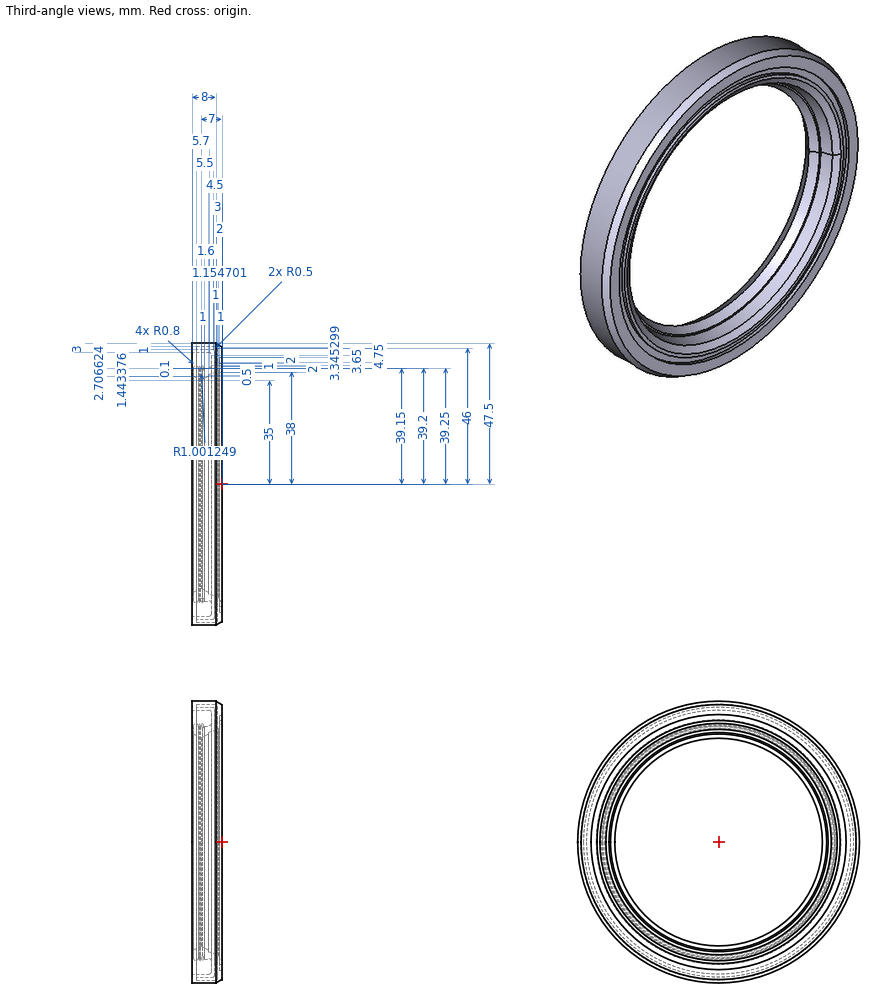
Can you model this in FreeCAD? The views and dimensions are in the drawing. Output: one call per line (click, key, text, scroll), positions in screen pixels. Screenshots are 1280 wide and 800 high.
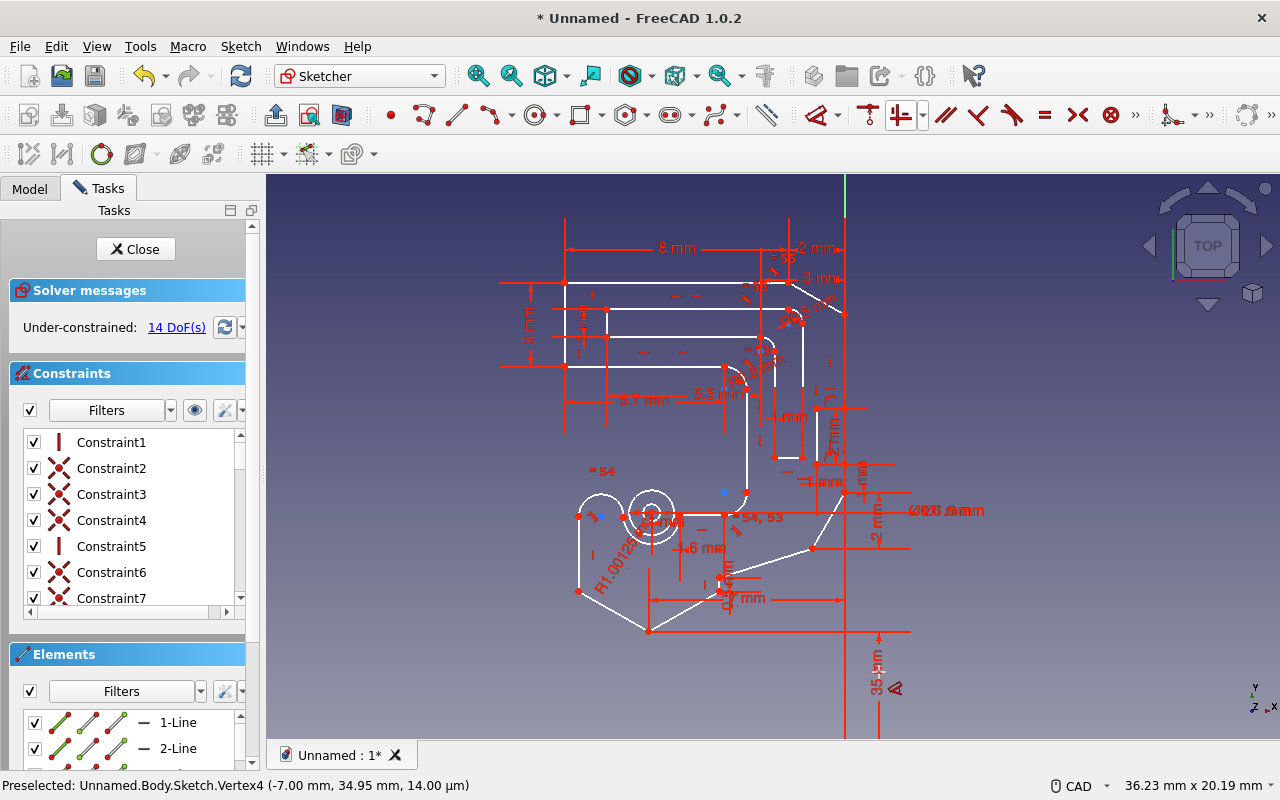
click(812, 549)
click(879, 630)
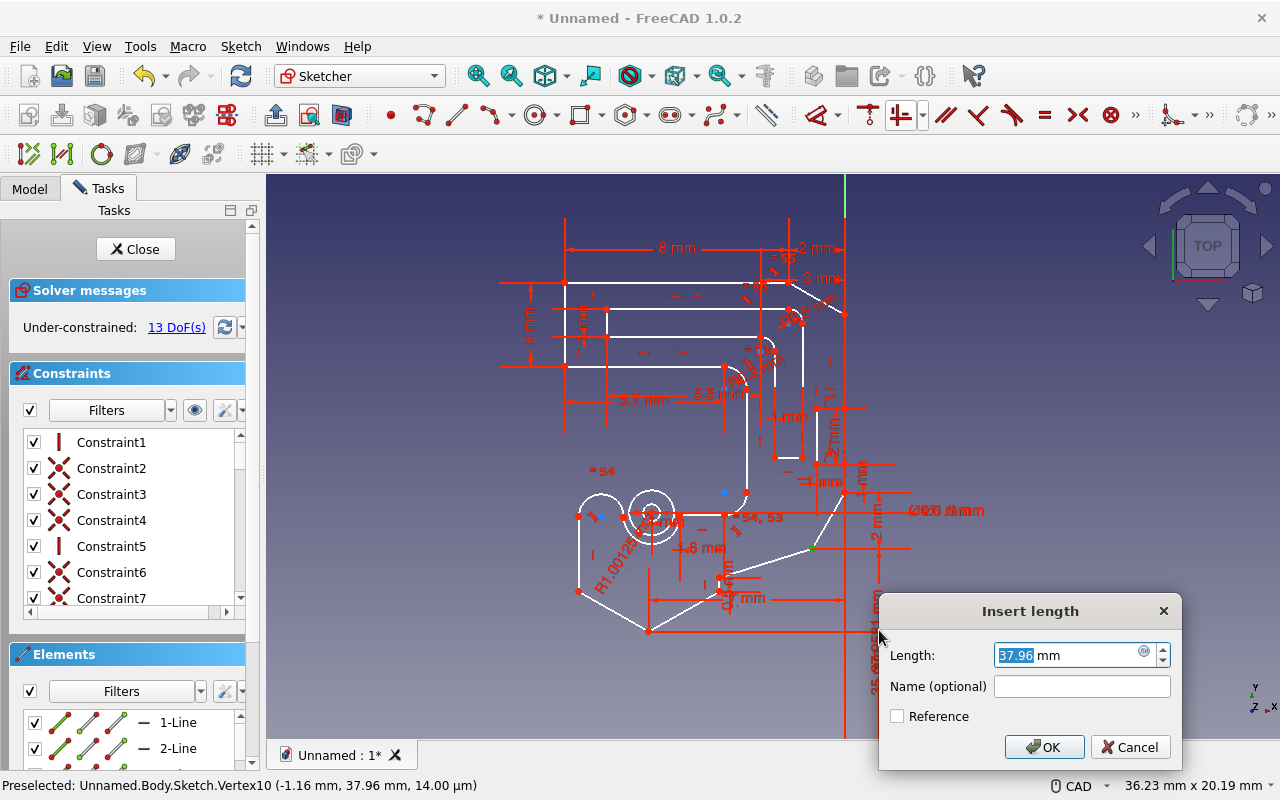
text(38)
key(Return)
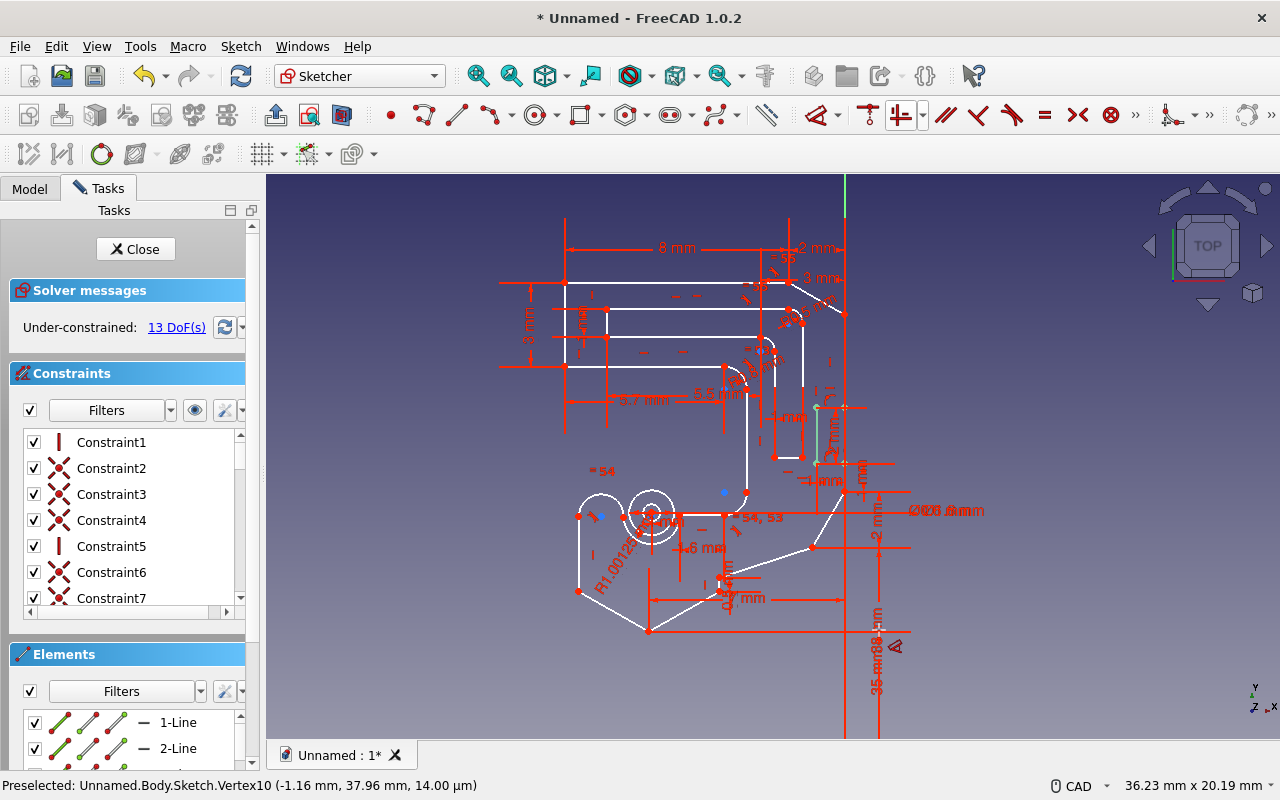
click(803, 323)
click(879, 606)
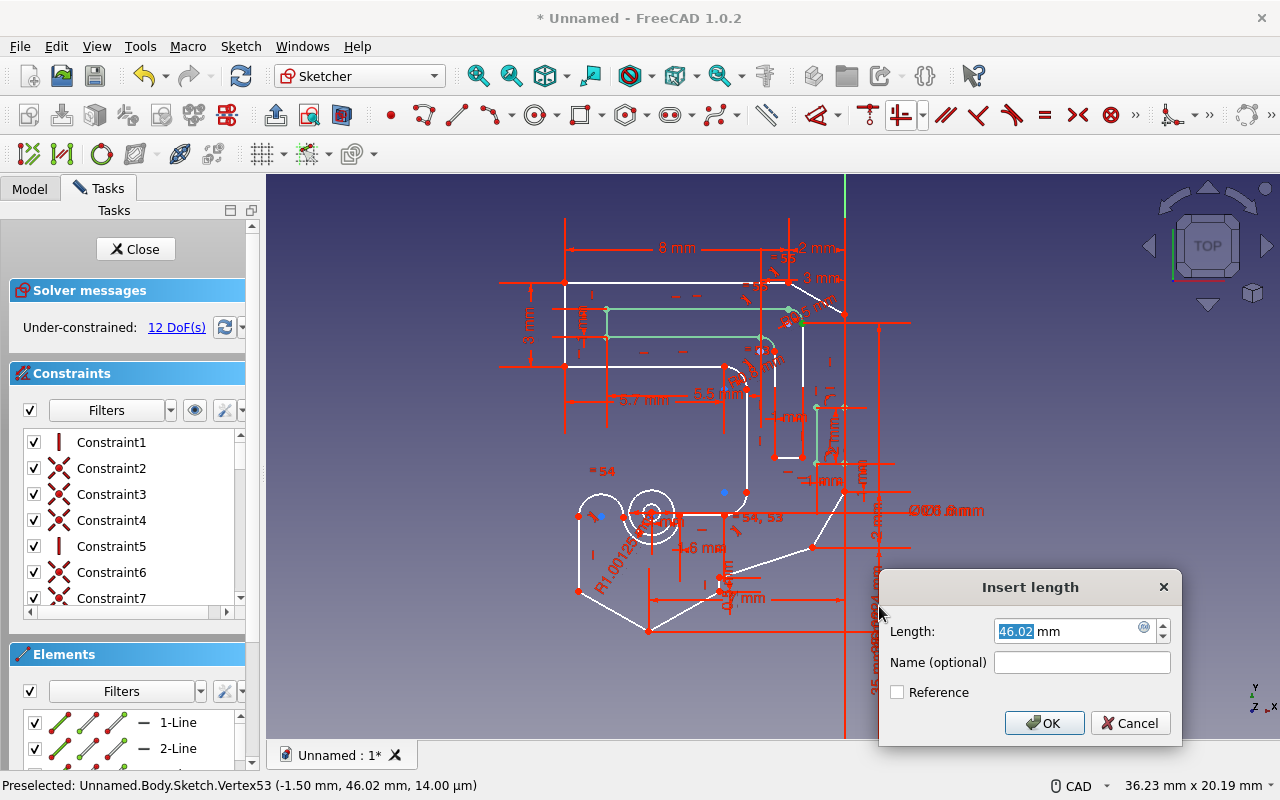
text(46)
key(Return)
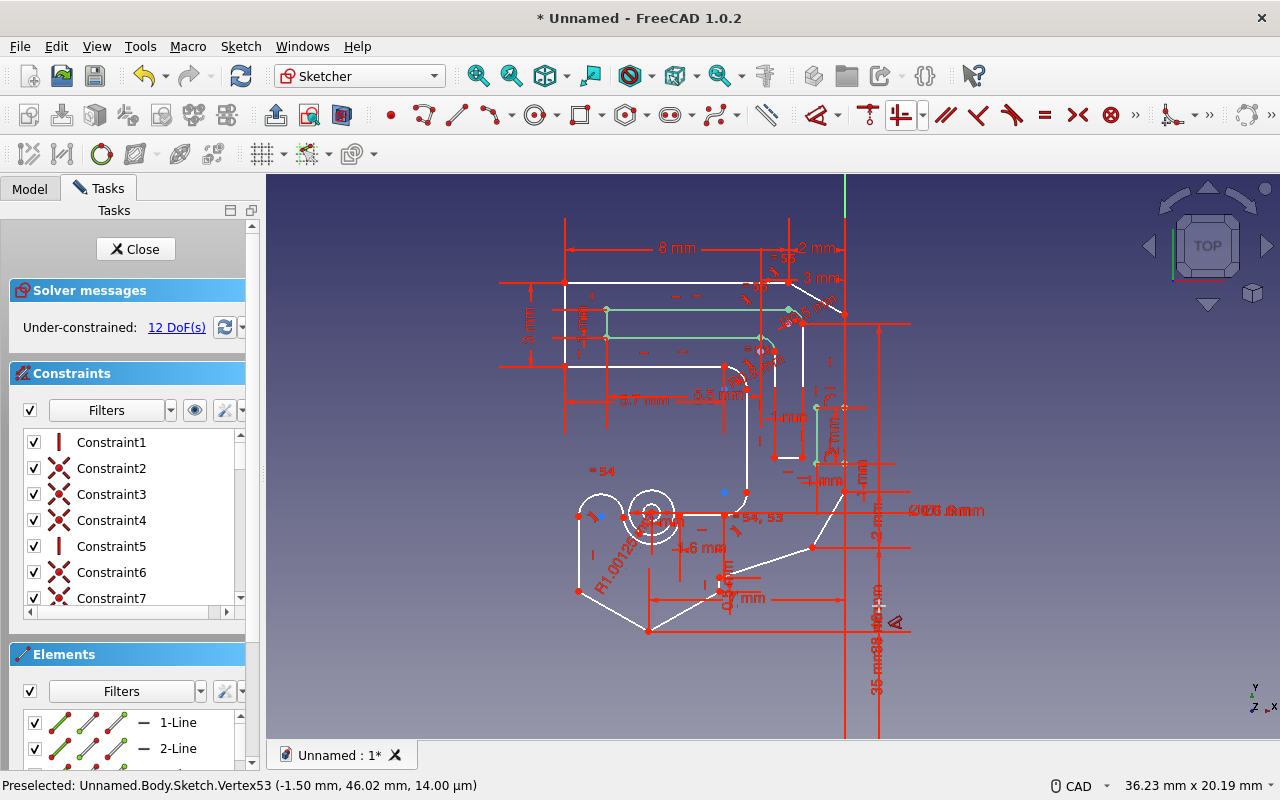
click(747, 420)
click(713, 441)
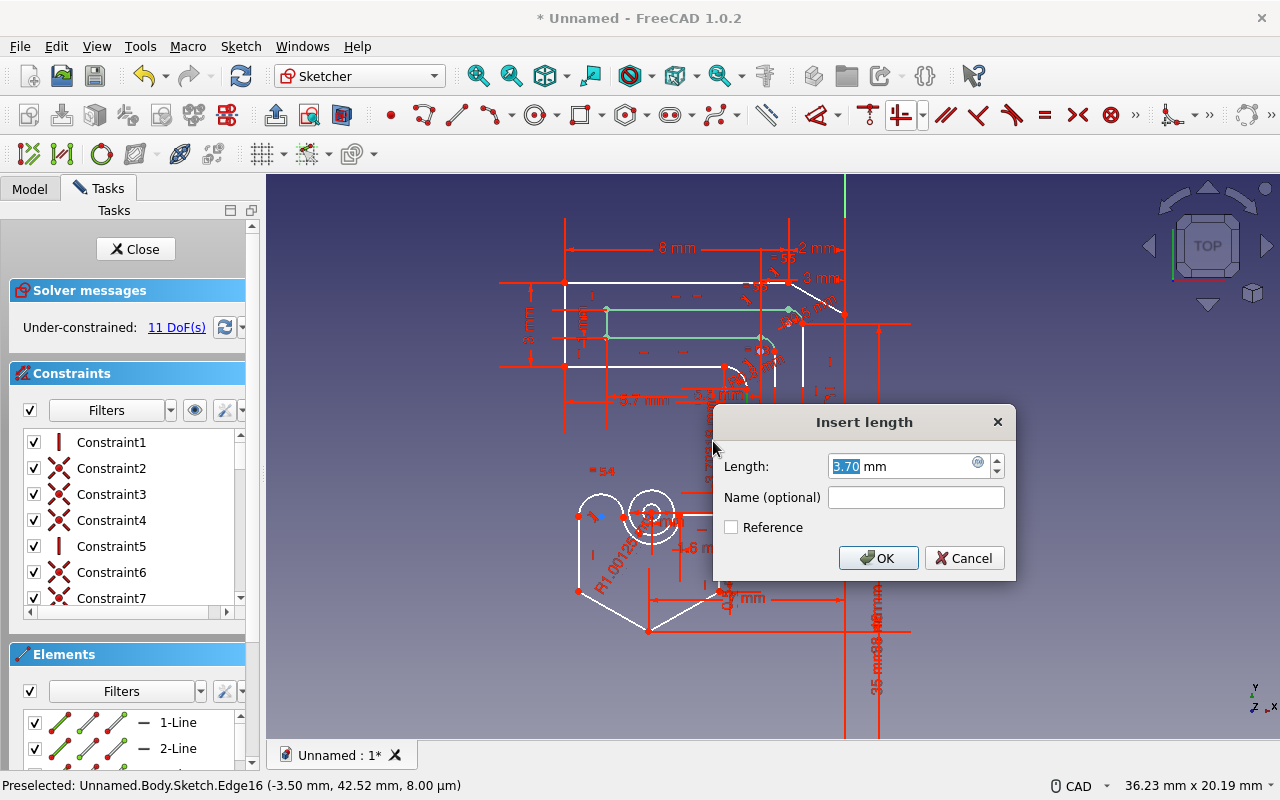
text(3.65)
key(Return)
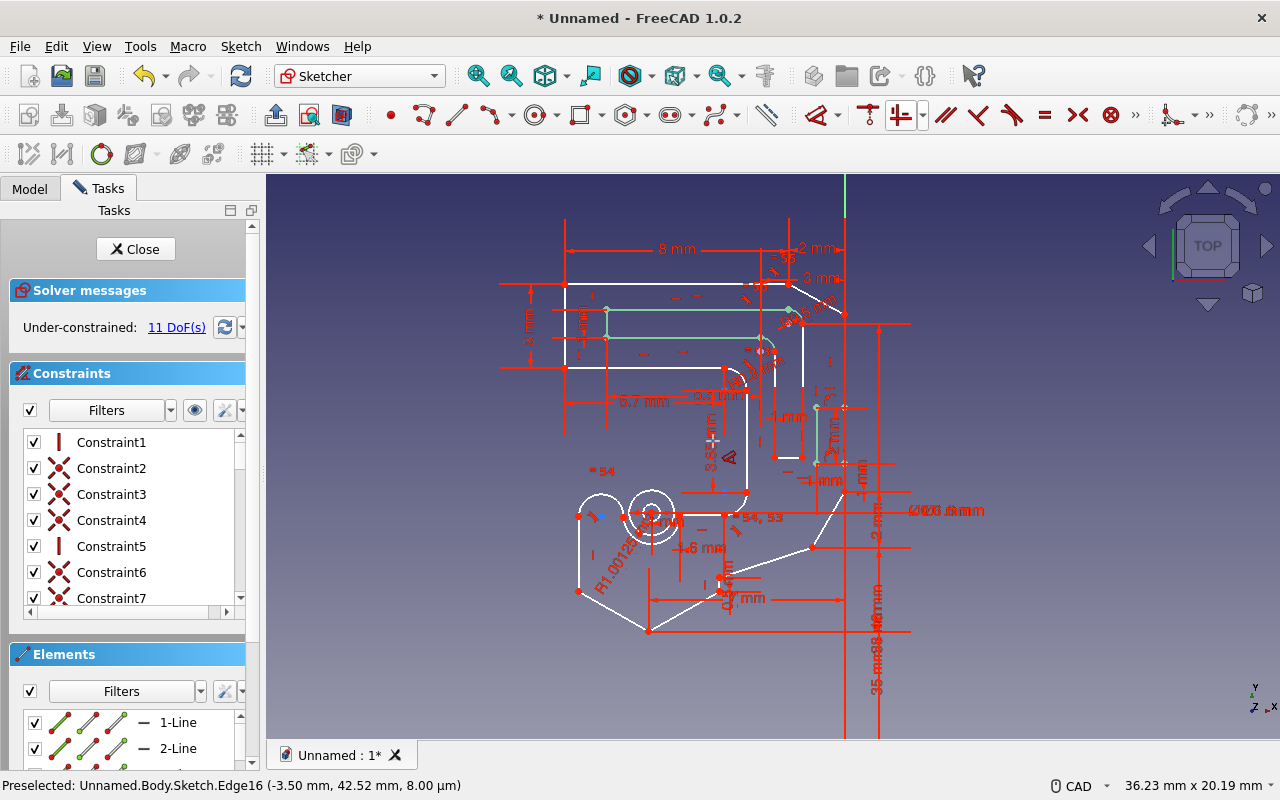
click(803, 364)
click(861, 391)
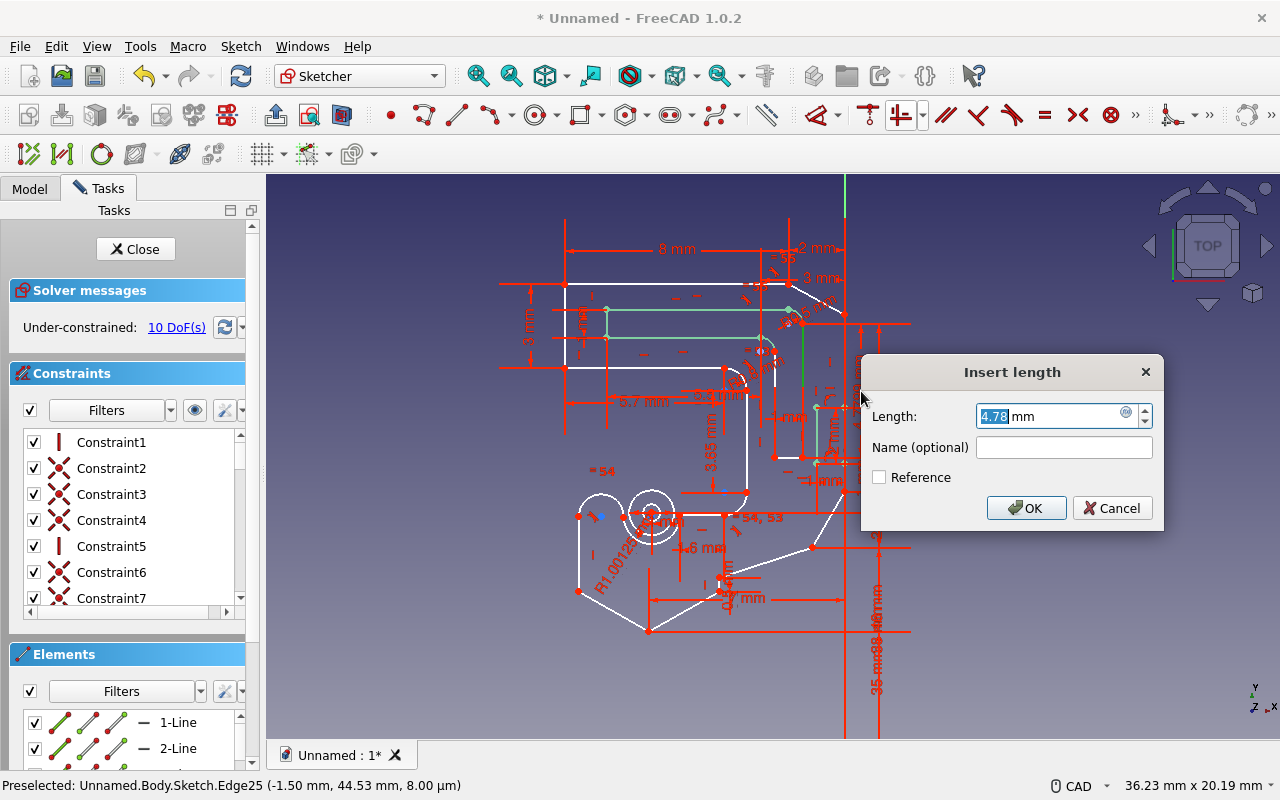
text(4.75)
key(Return)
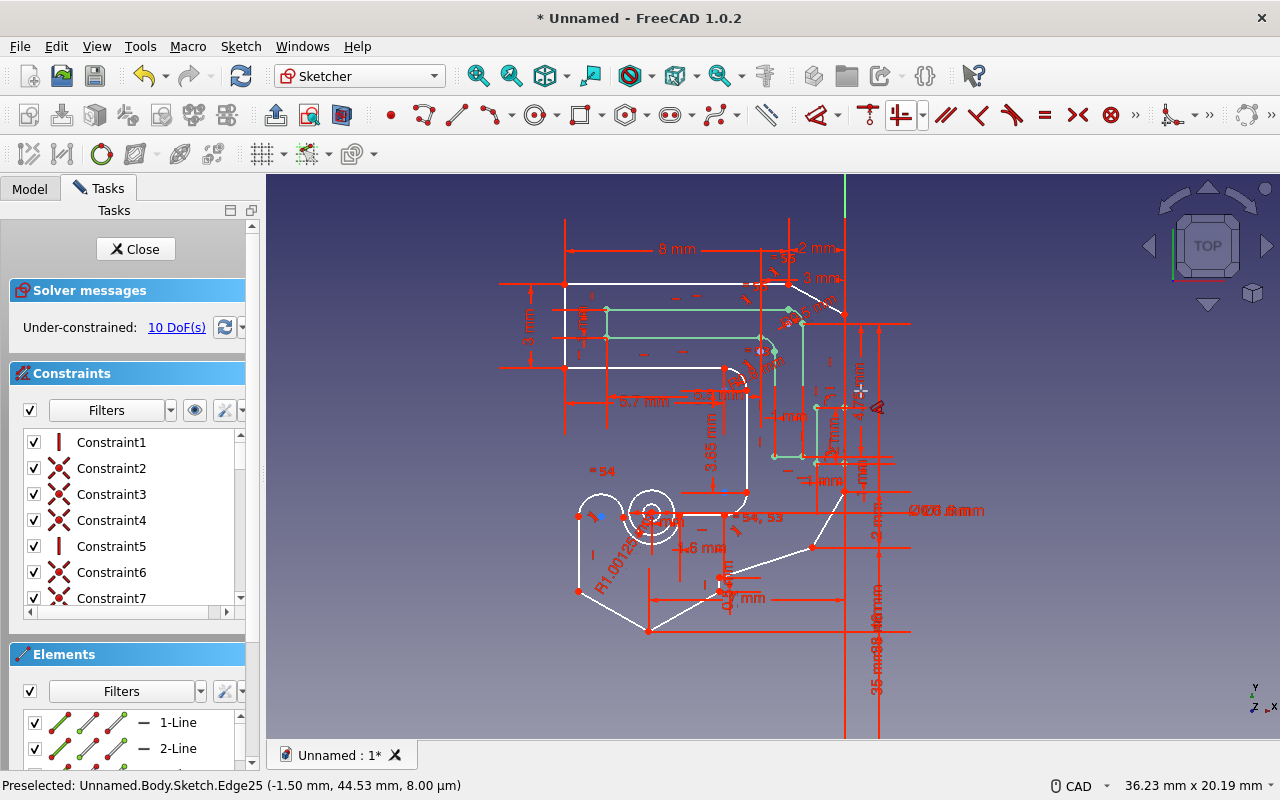
click(719, 592)
click(826, 558)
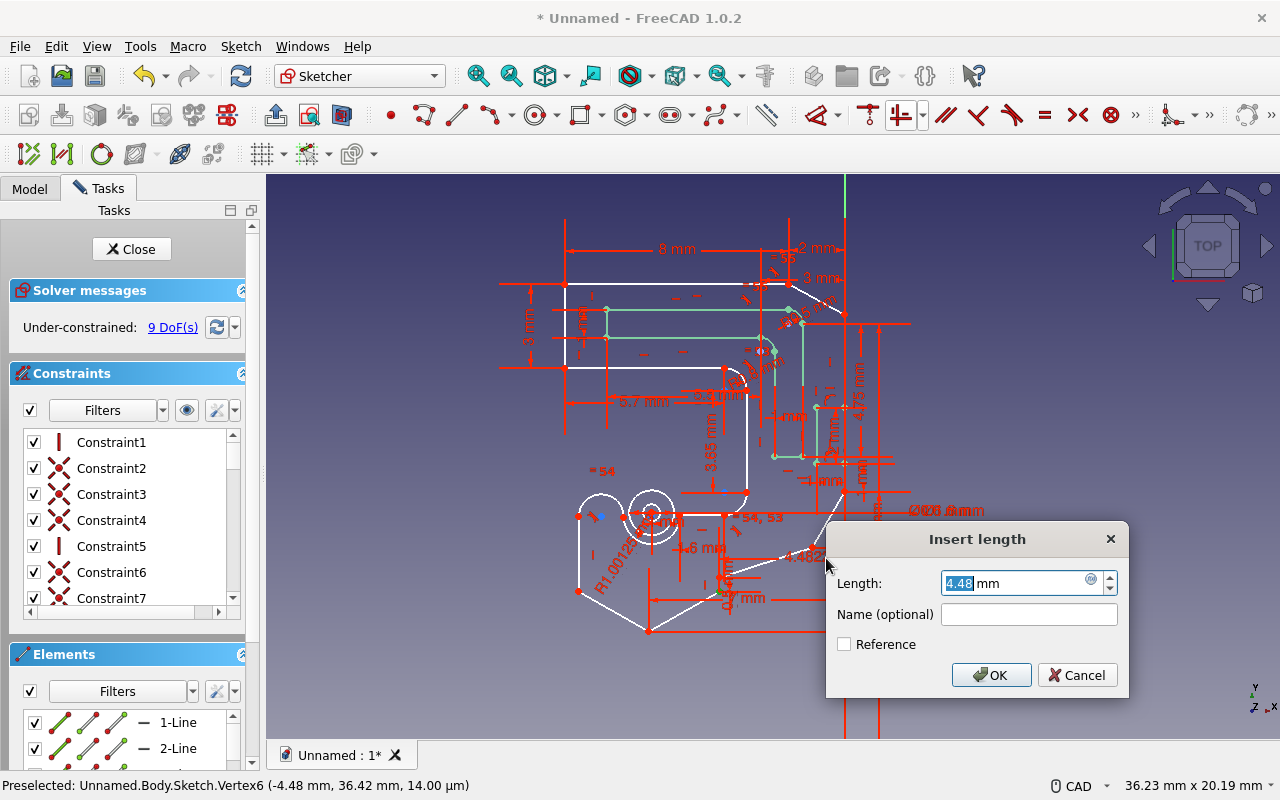
text(4.5)
key(Return)